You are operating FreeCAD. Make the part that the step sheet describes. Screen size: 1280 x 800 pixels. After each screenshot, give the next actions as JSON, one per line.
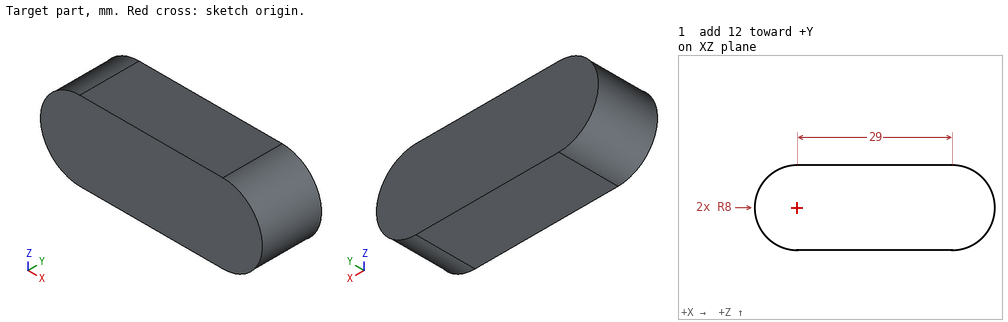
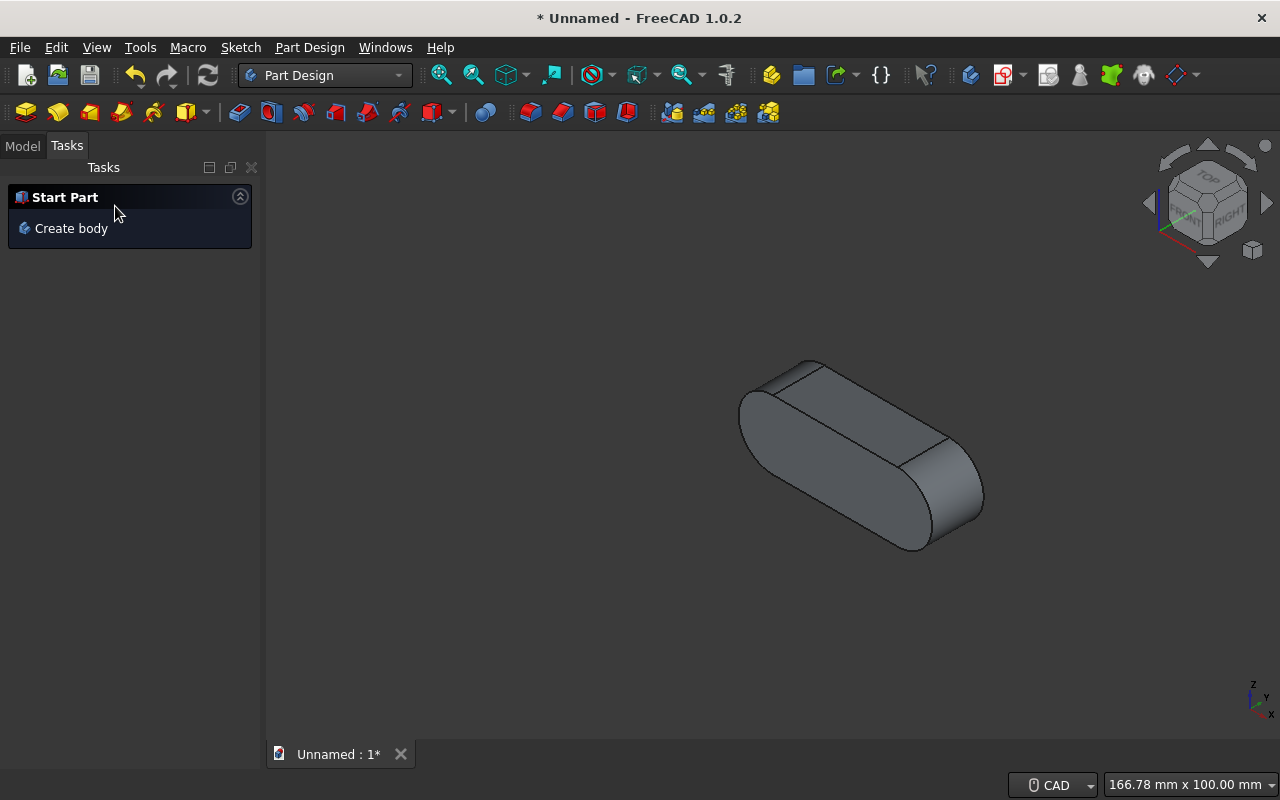
{"action": "left_click", "coordinate": [442, 76]}